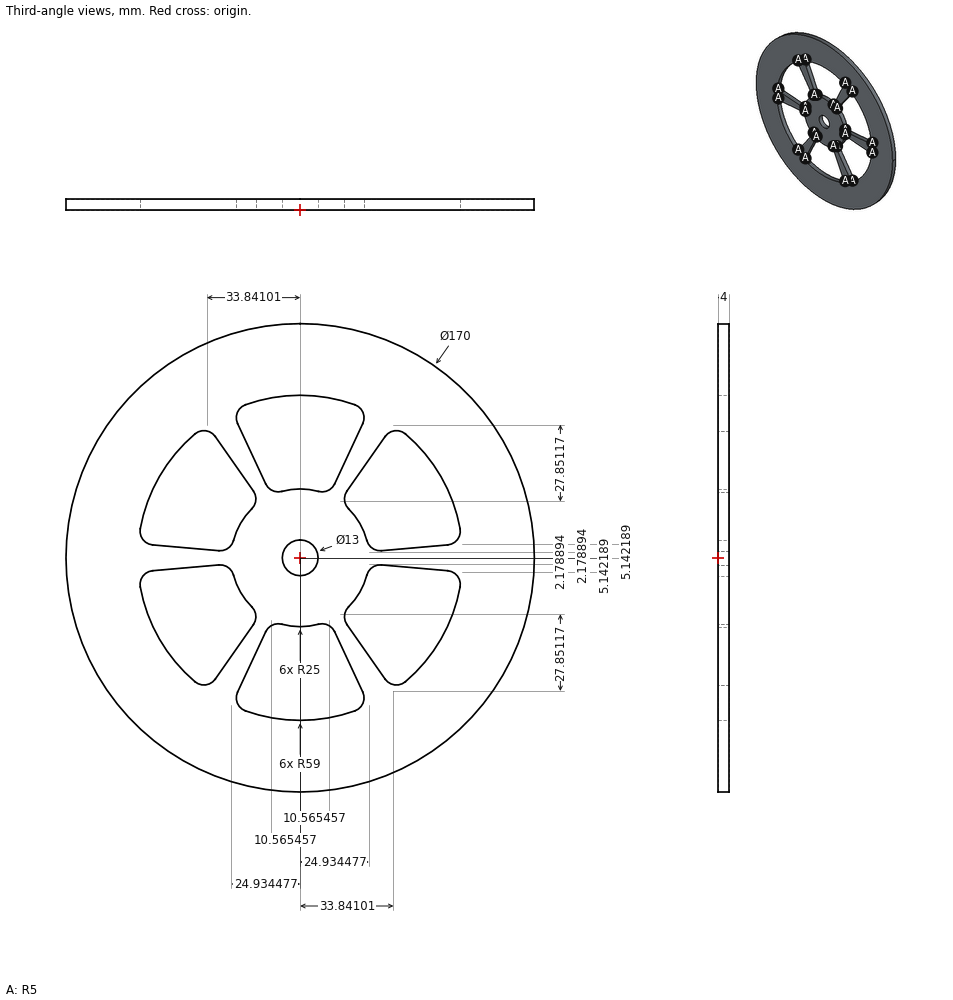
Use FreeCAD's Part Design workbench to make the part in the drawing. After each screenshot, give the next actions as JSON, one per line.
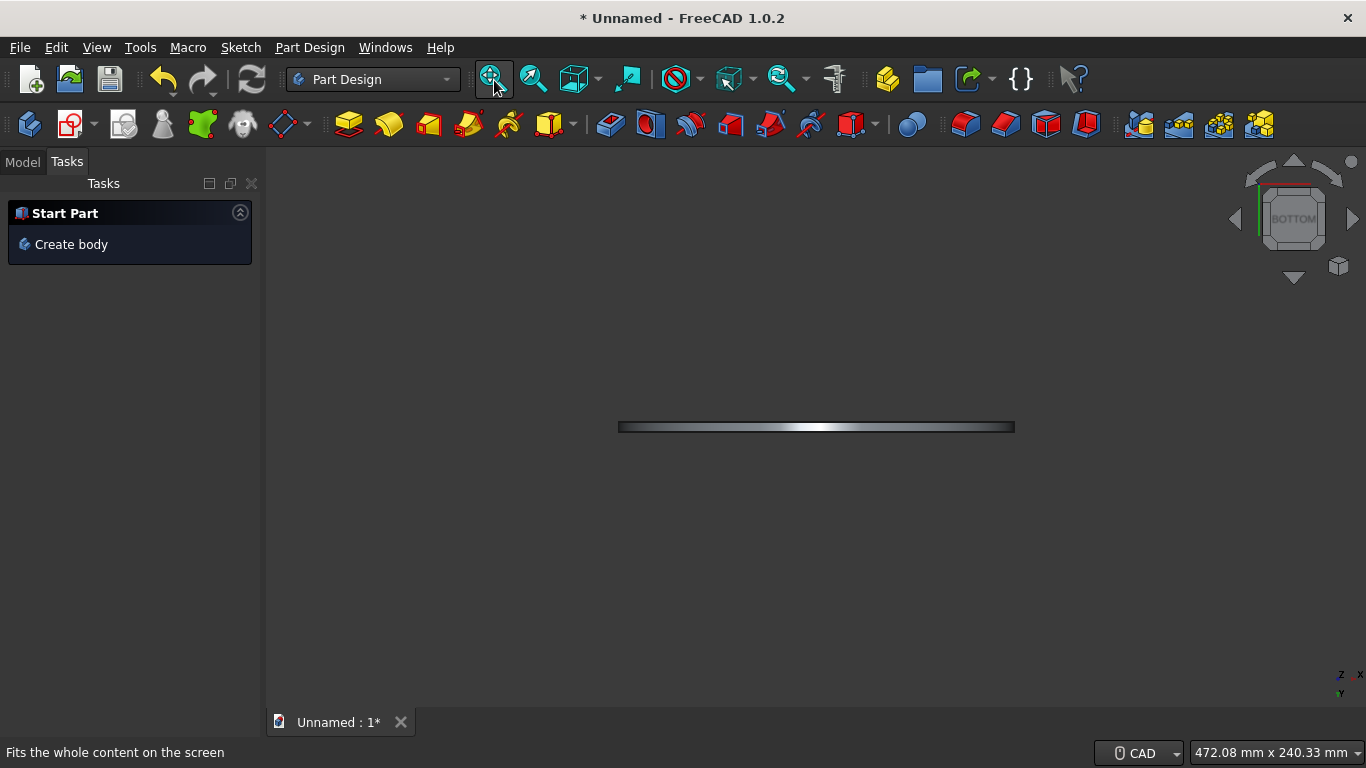
{"action": "key", "text": "4"}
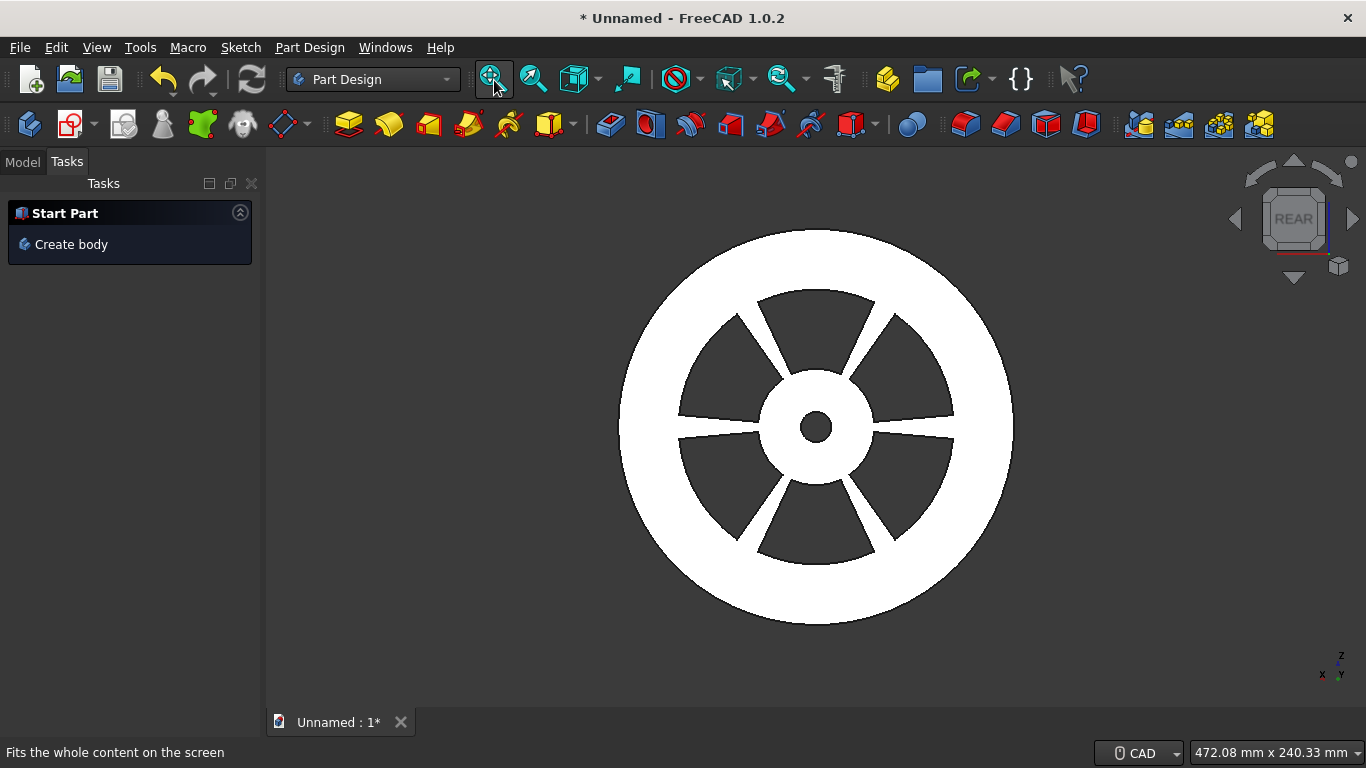
{"action": "scroll", "coordinate": [841, 373], "scroll_direction": "up", "scroll_amount": 8}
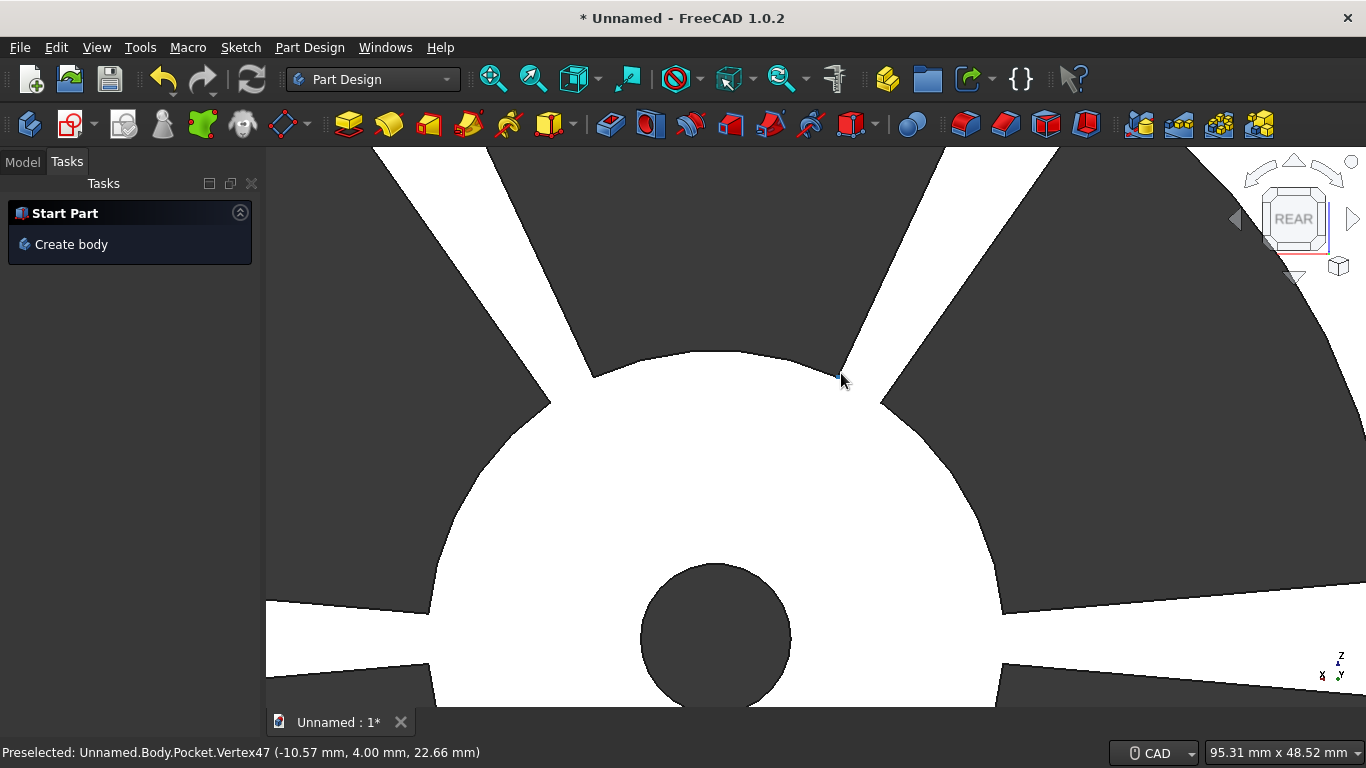
{"action": "left_click", "coordinate": [494, 80]}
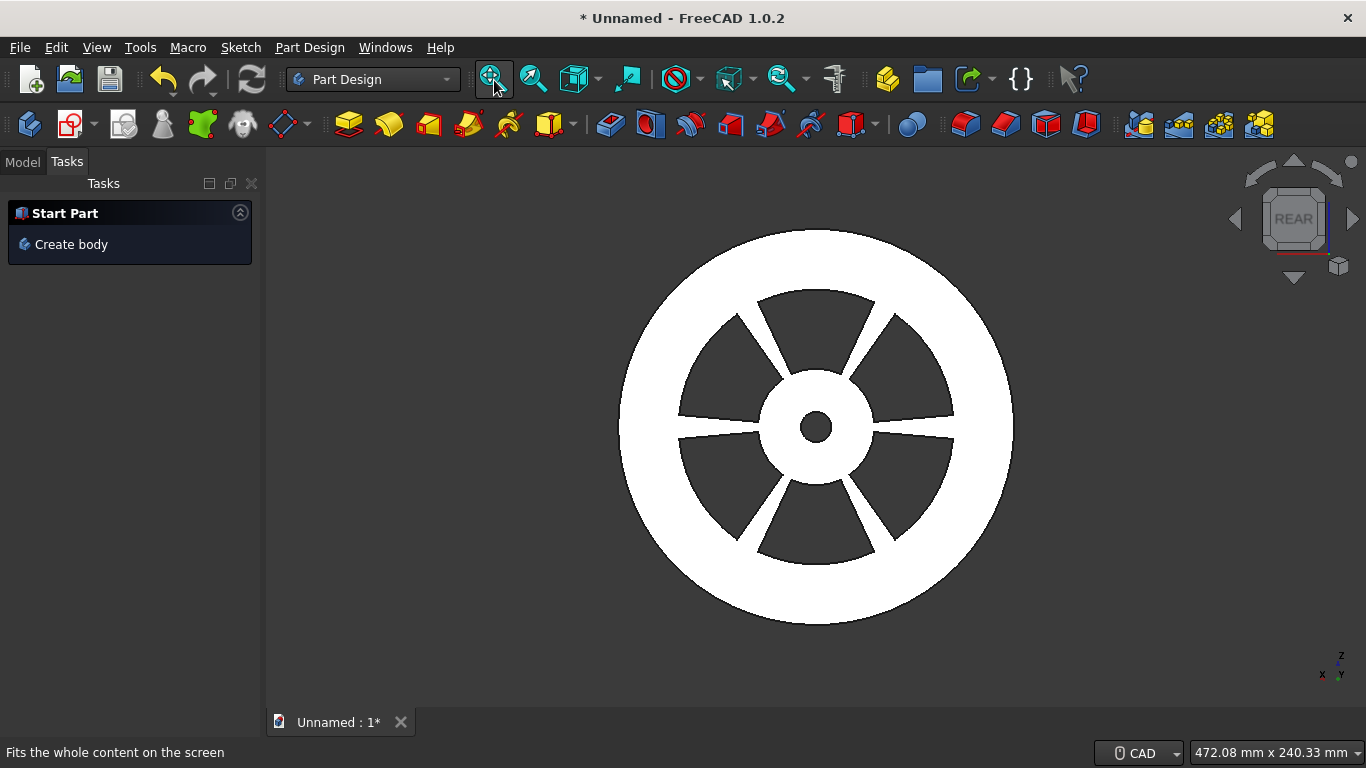
{"action": "key", "text": "6"}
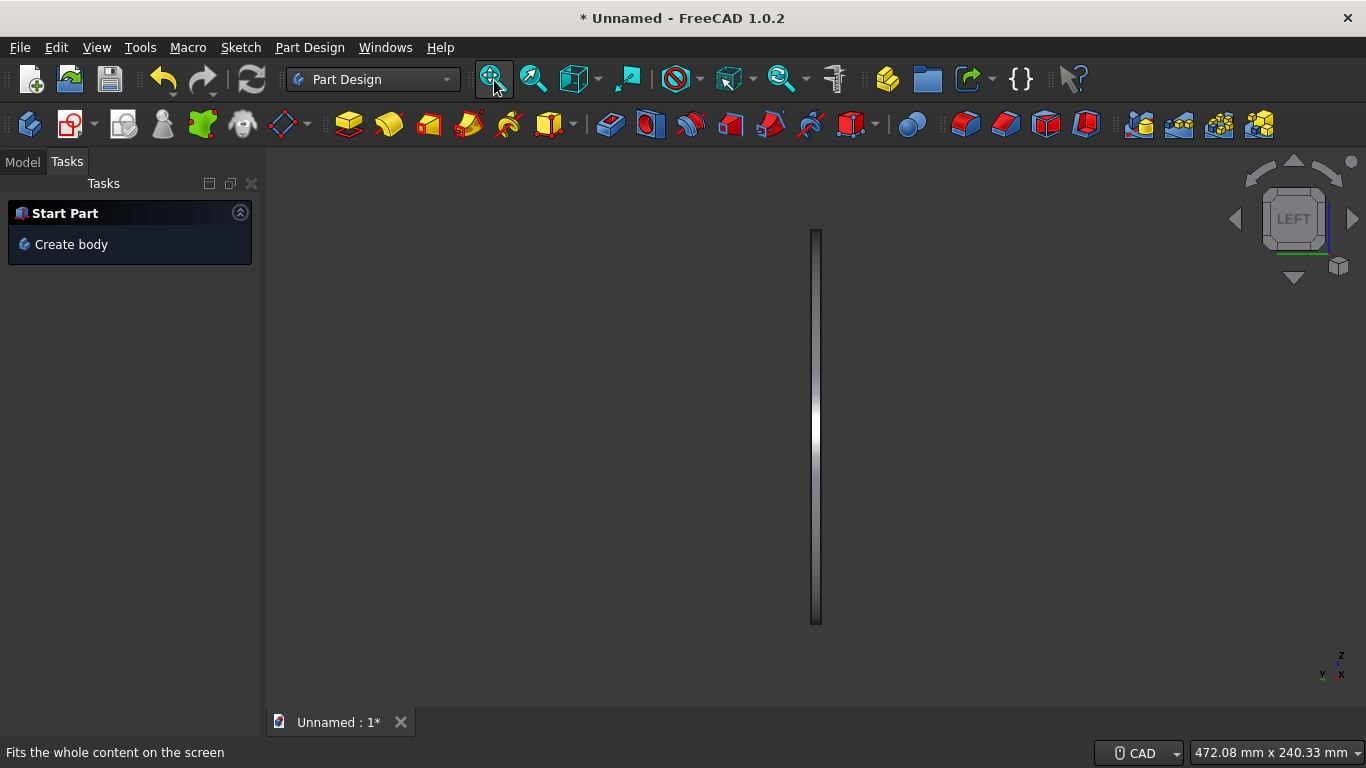
{"action": "scroll", "coordinate": [816, 373], "scroll_direction": "up", "scroll_amount": 8}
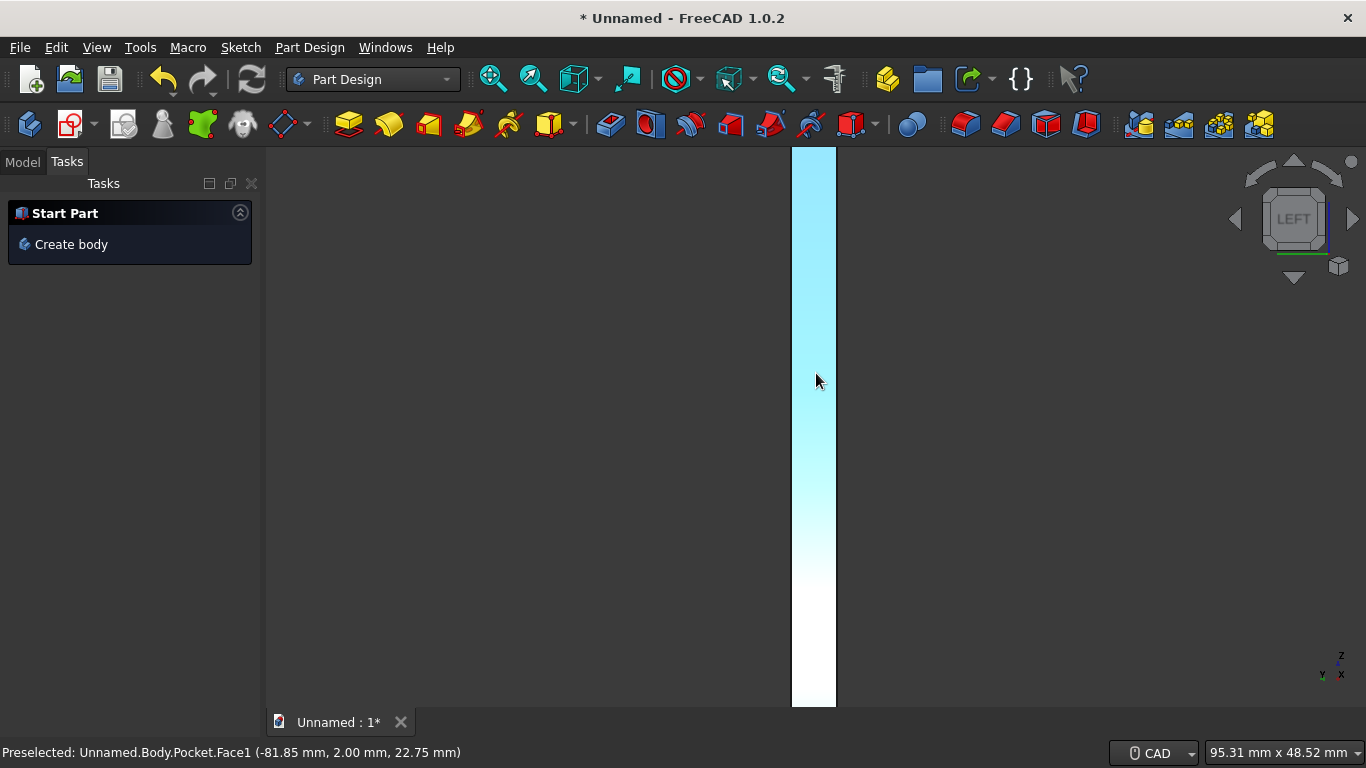
{"action": "left_click", "coordinate": [494, 80]}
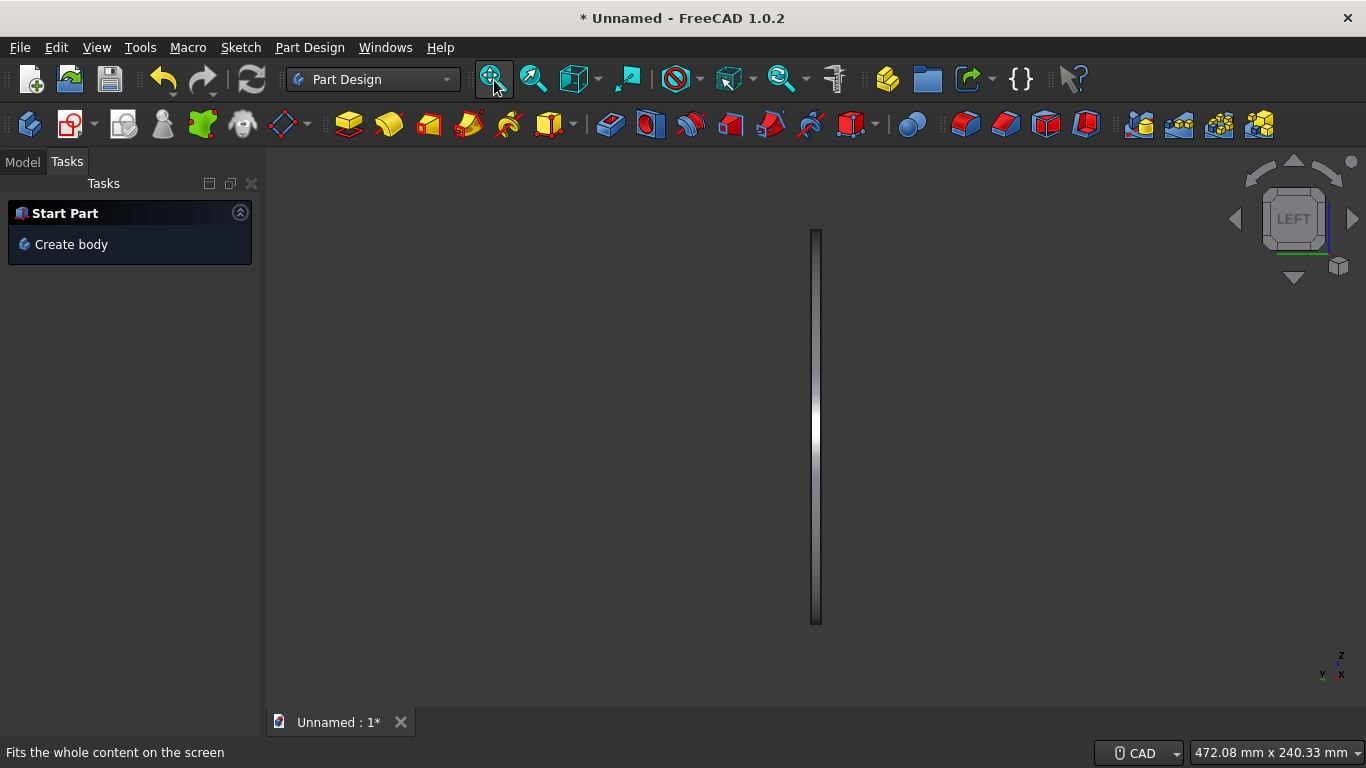
{"action": "key", "text": "v 3"}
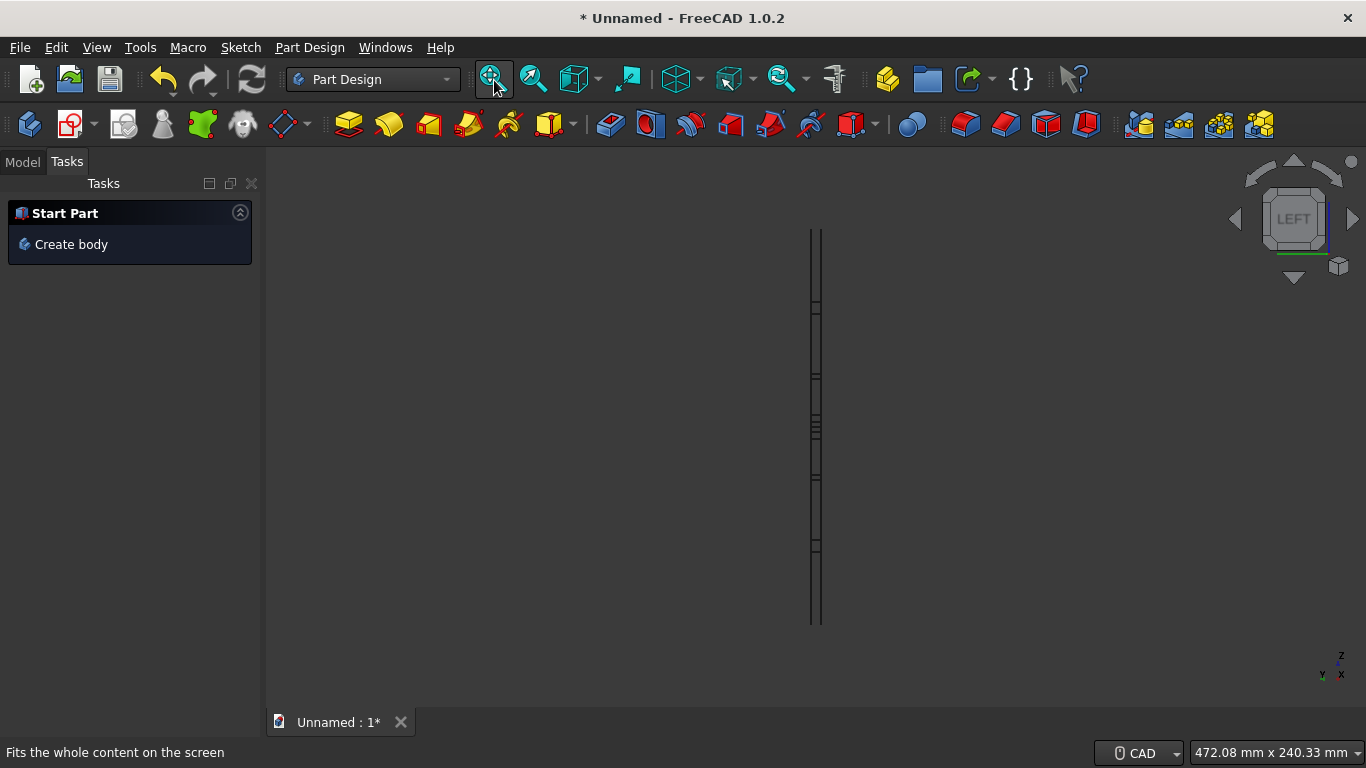
{"action": "key", "text": "0"}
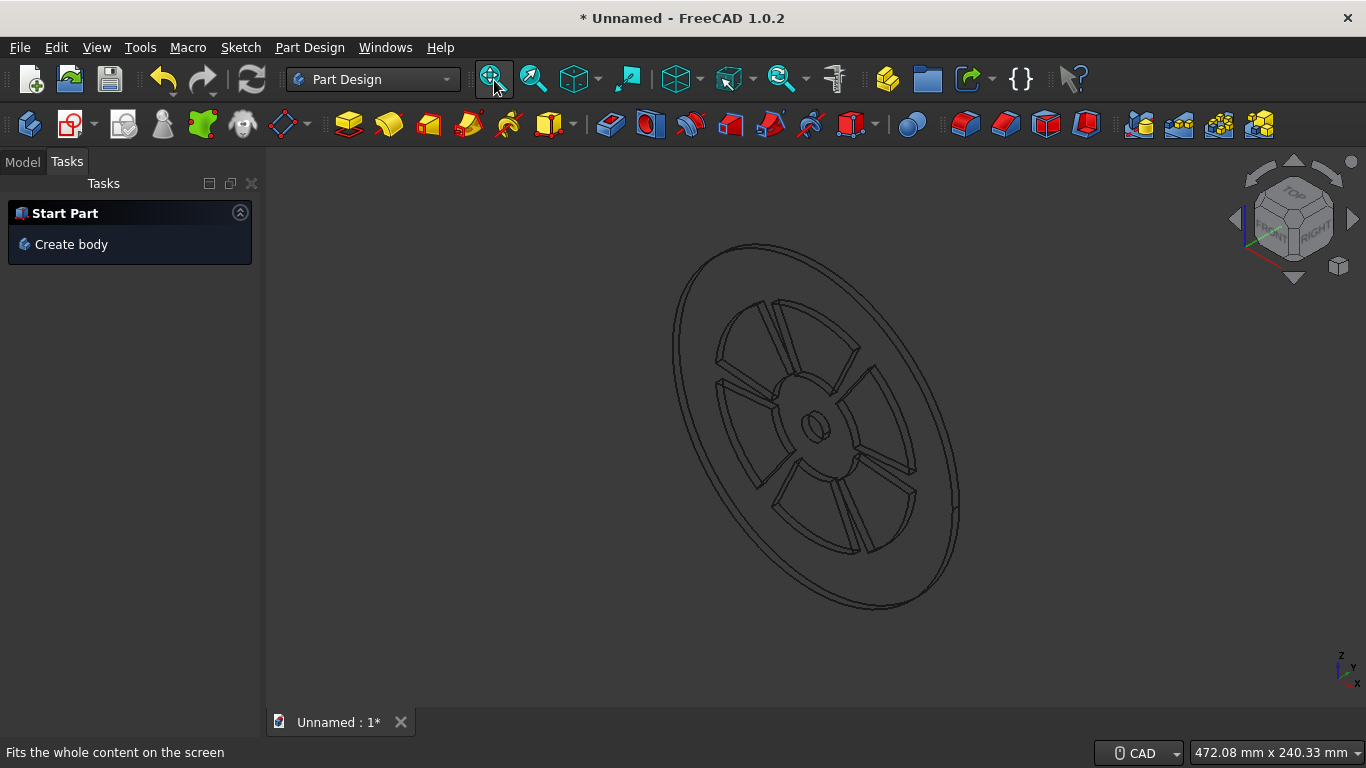
{"action": "scroll", "coordinate": [798, 373], "scroll_direction": "up", "scroll_amount": 8}